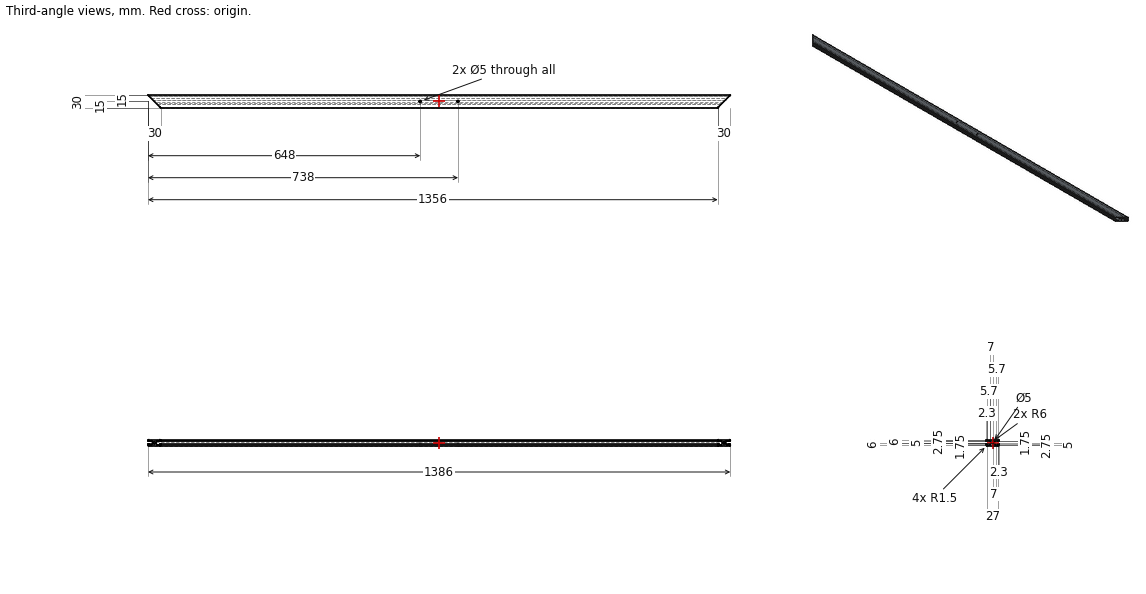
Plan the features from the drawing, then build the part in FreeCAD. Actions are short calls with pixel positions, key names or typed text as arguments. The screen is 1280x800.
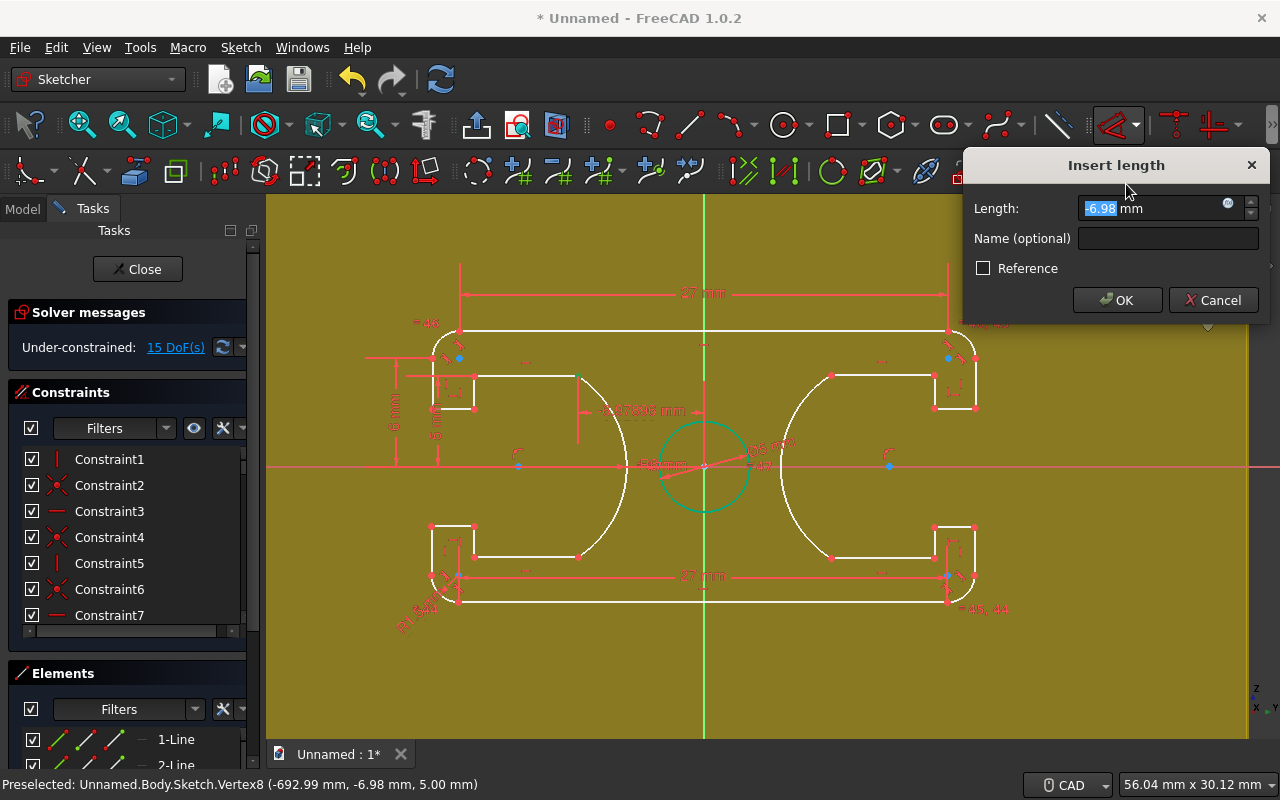
text(-7)
key(Return)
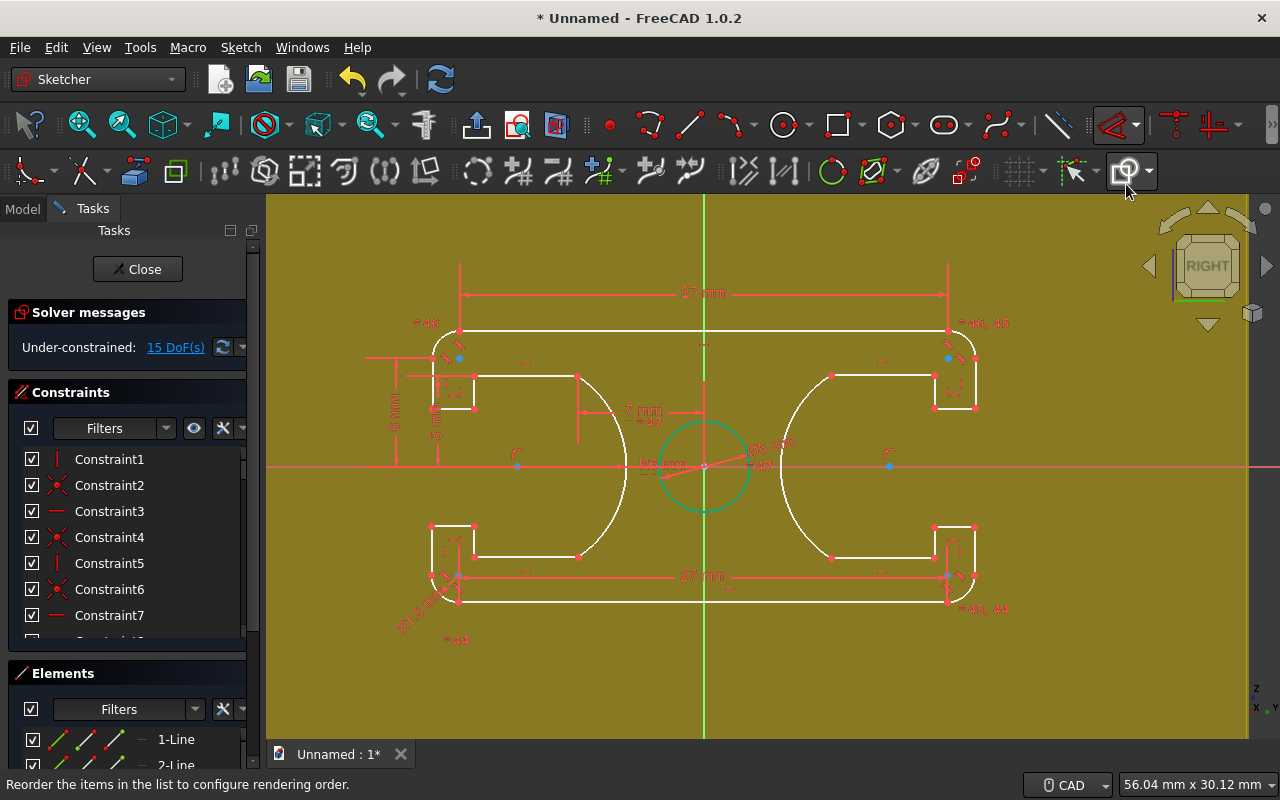
click(578, 557)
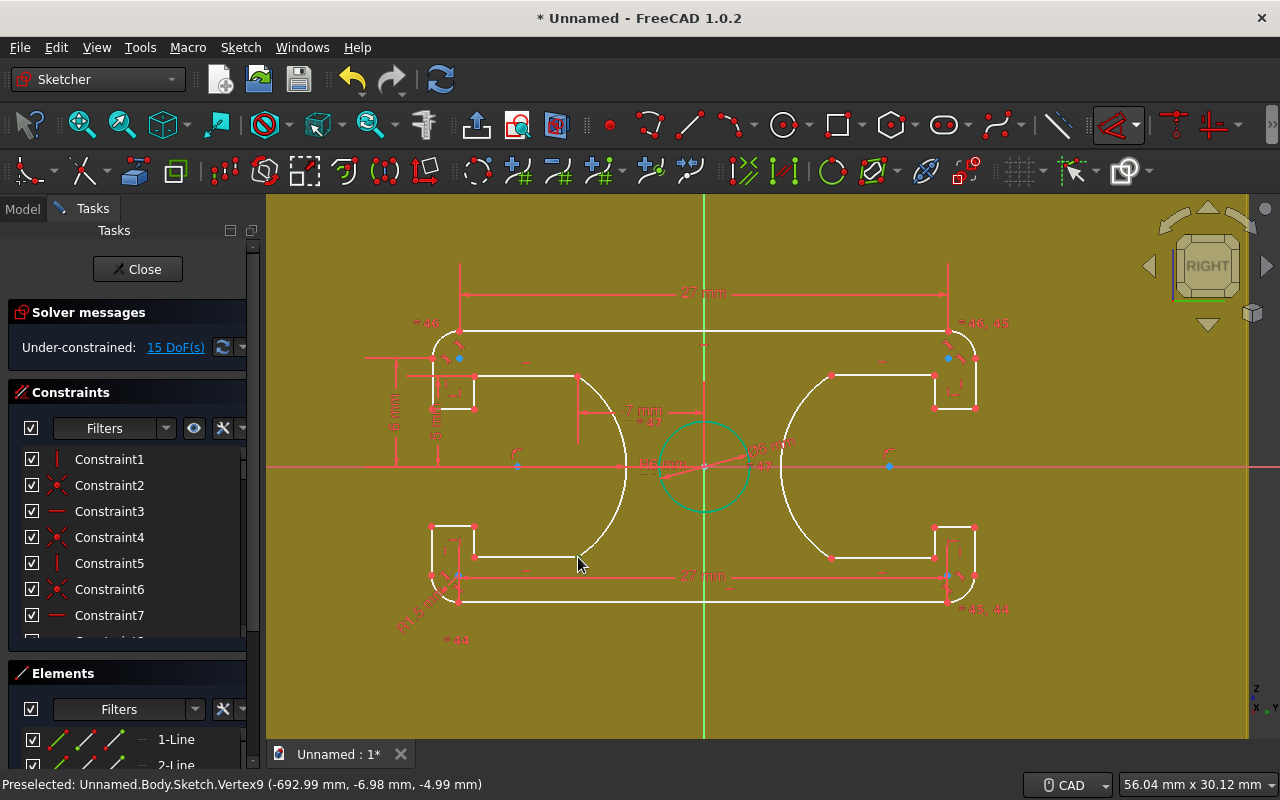
key(l)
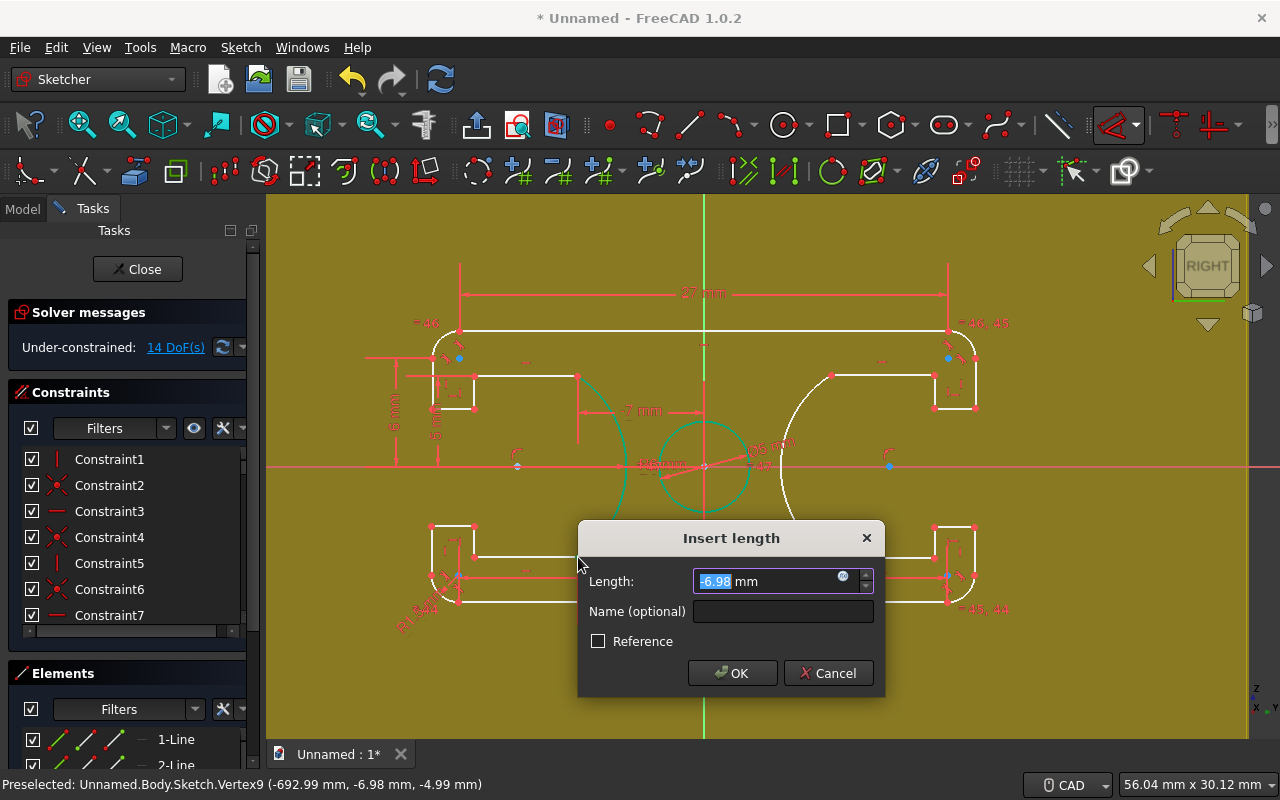
text(-7)
key(Return)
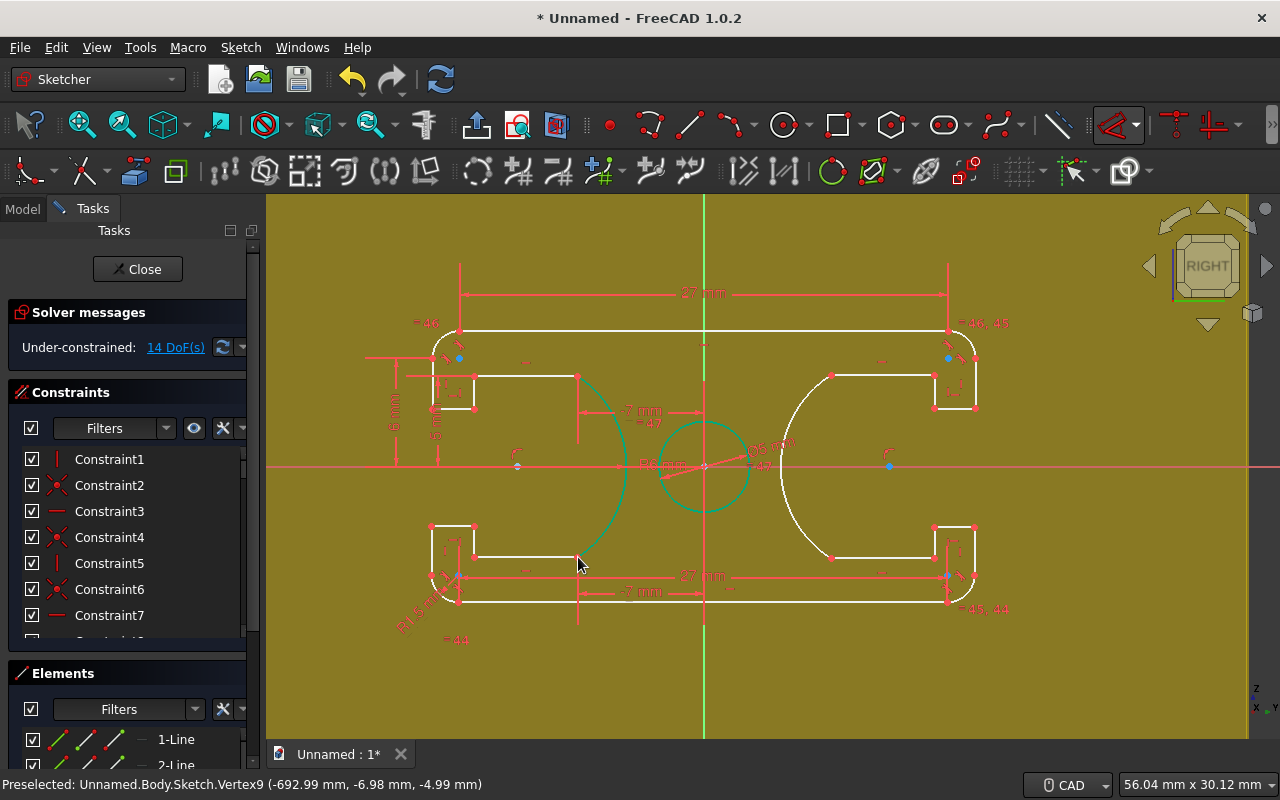
click(432, 575)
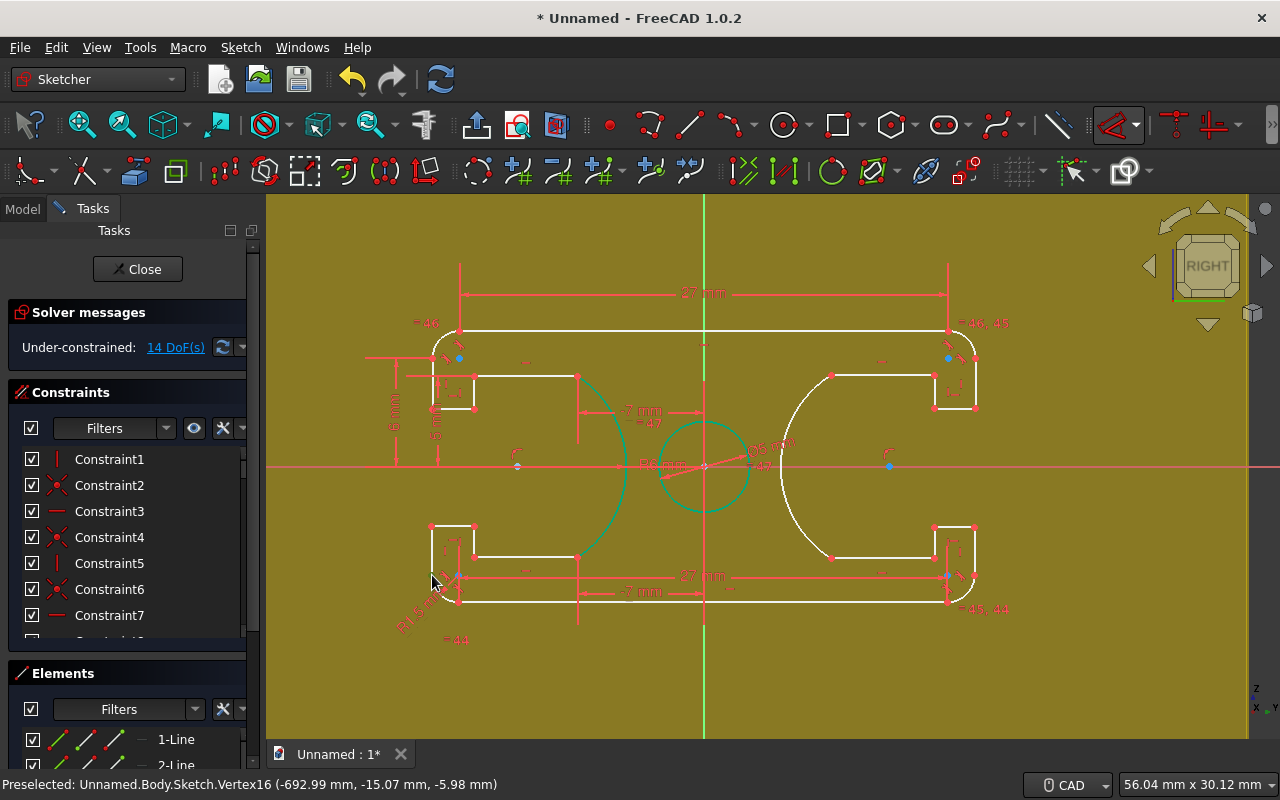
click(1138, 126)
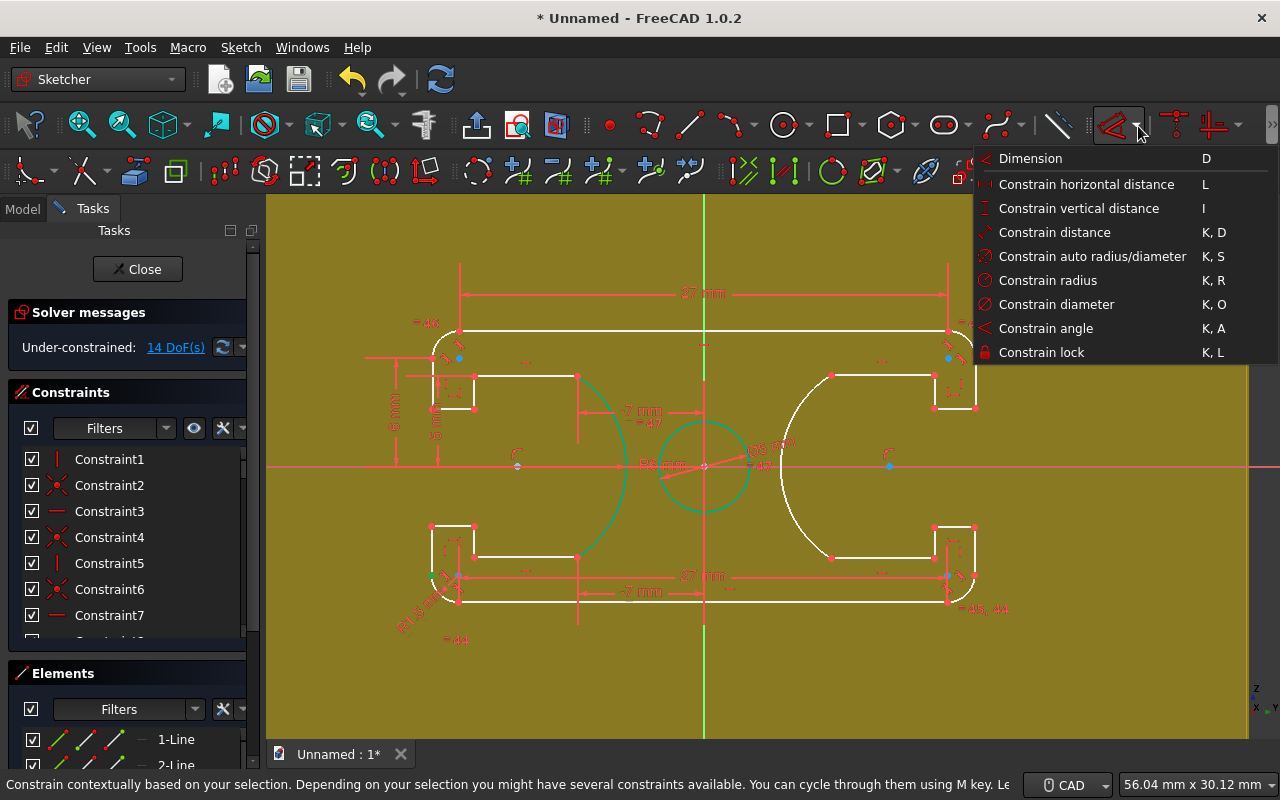
click(1126, 208)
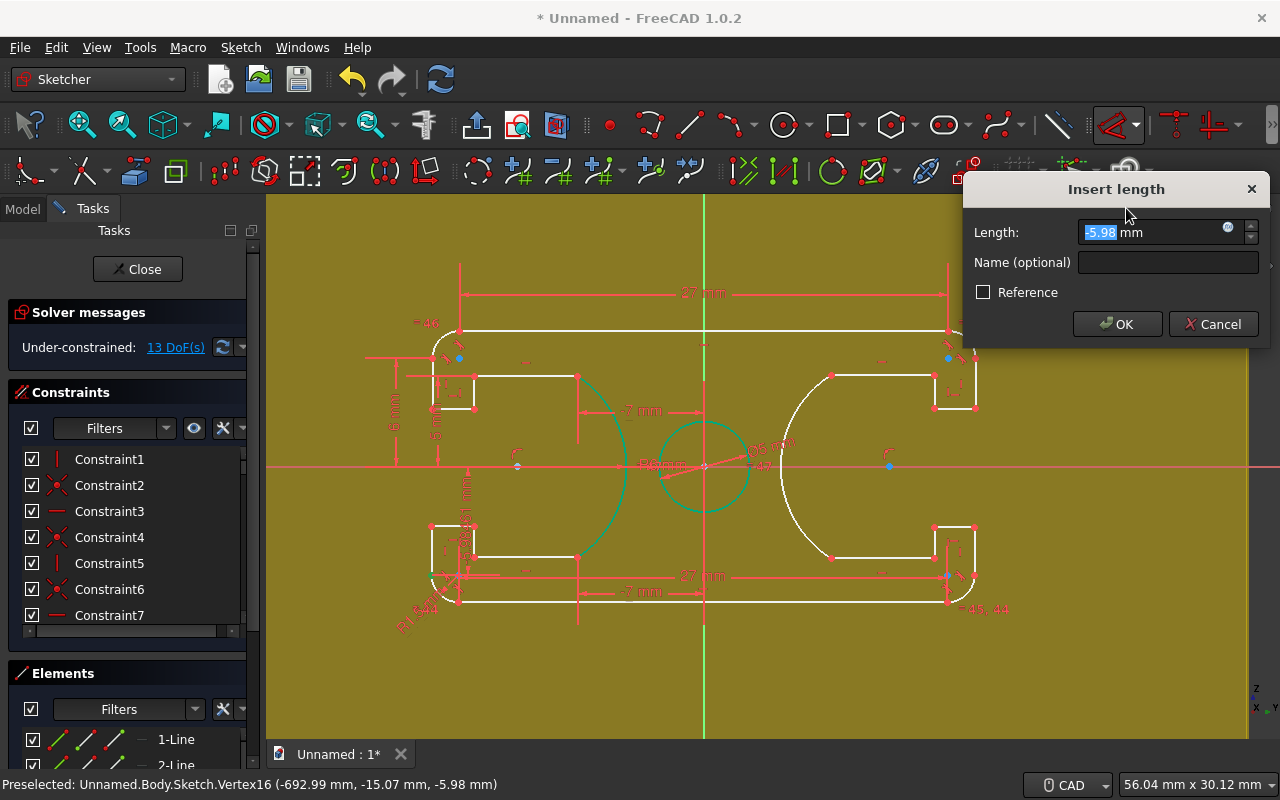
text(-6)
key(Return)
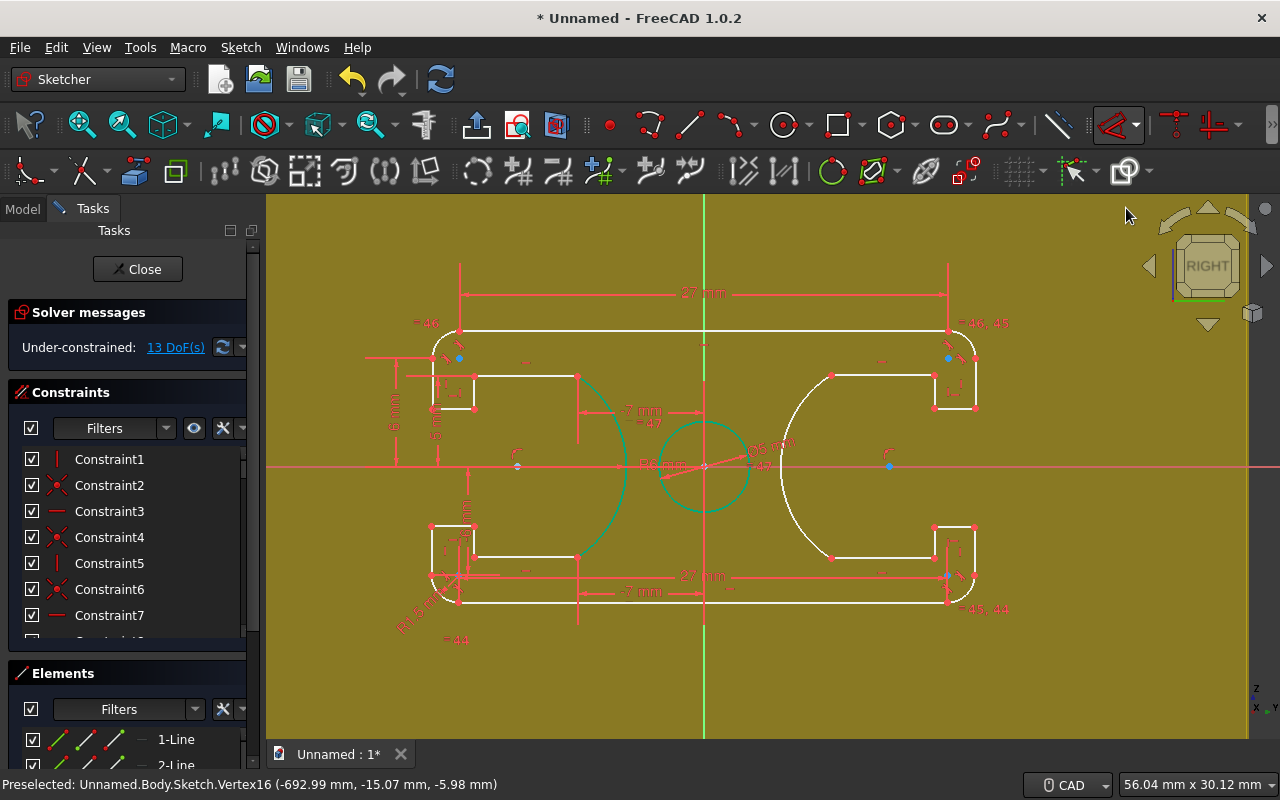
click(935, 558)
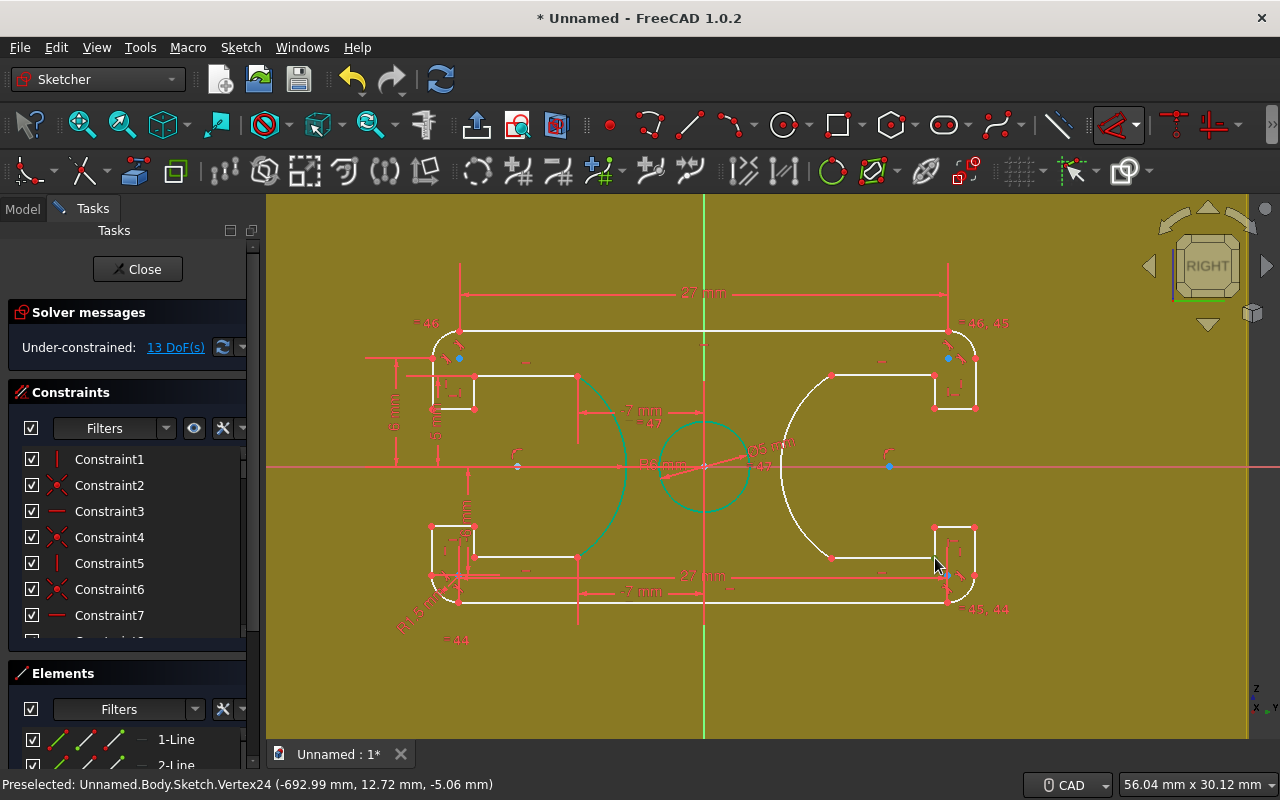
key(i)